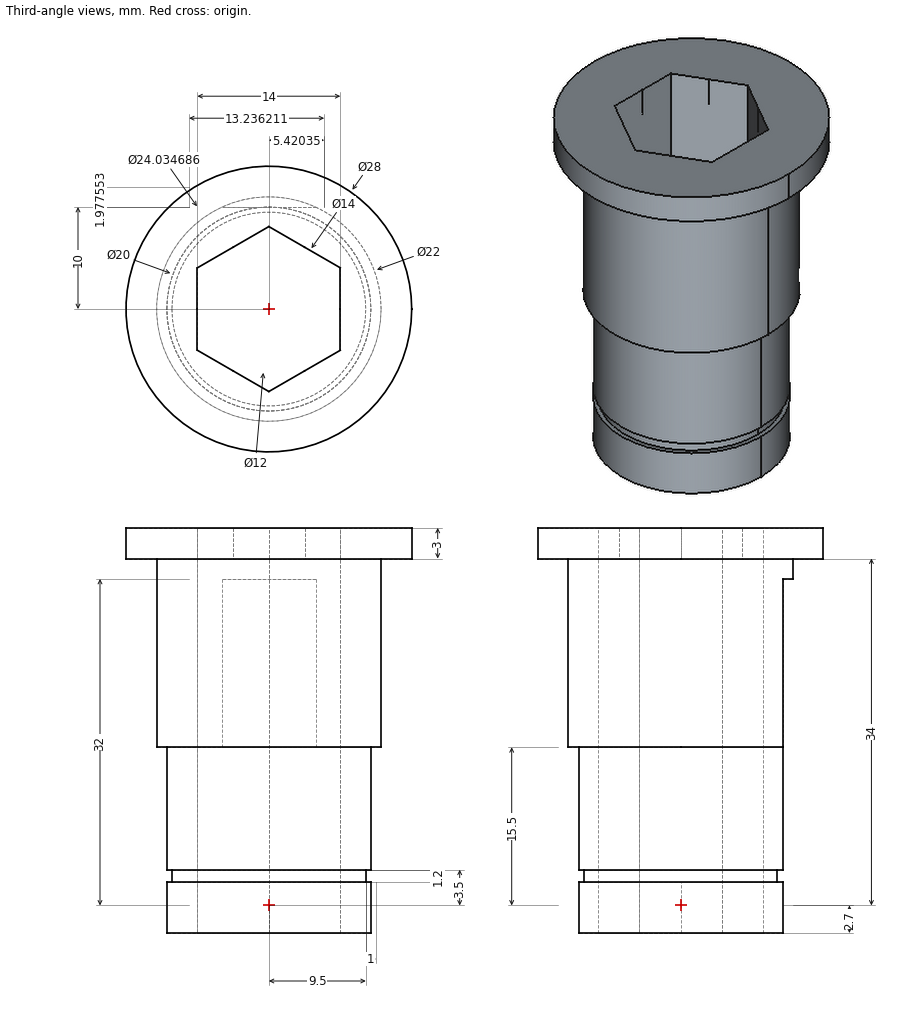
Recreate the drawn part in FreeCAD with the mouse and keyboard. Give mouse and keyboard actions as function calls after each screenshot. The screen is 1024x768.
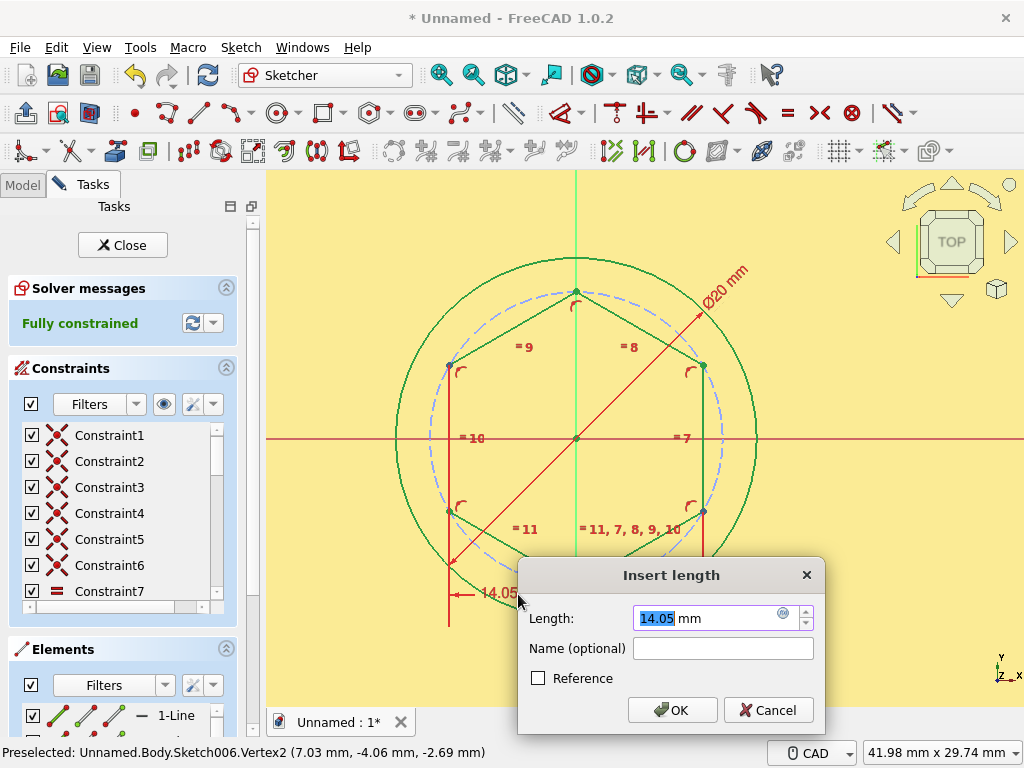
text(14)
key(Return)
key(Escape)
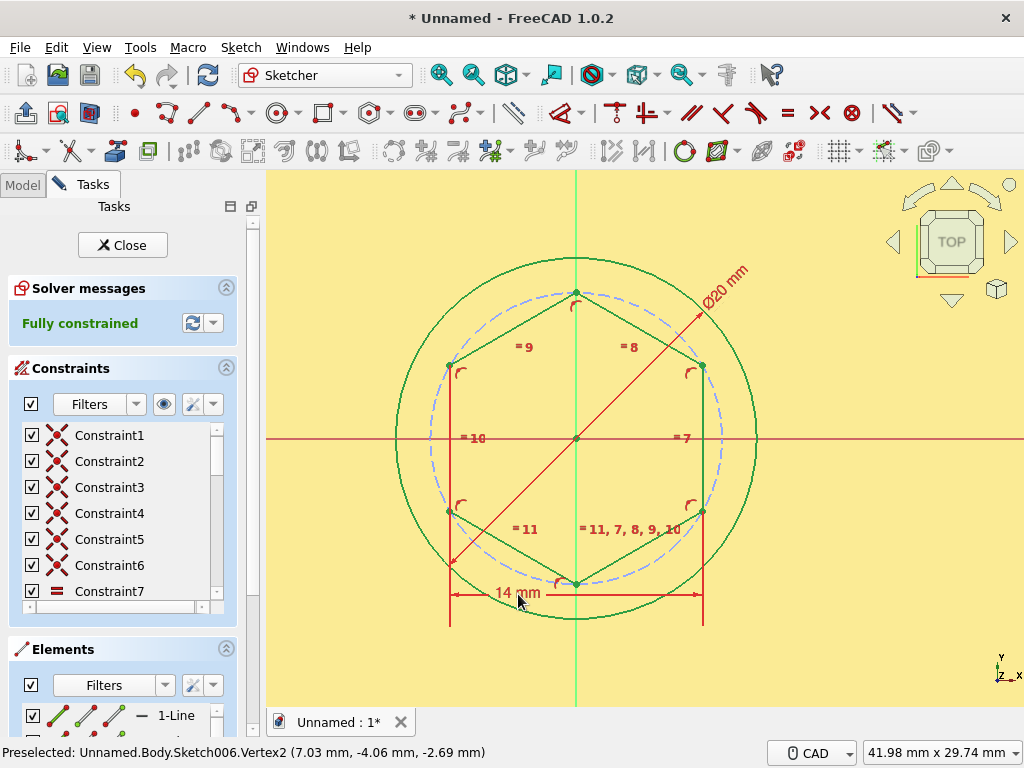
click(123, 245)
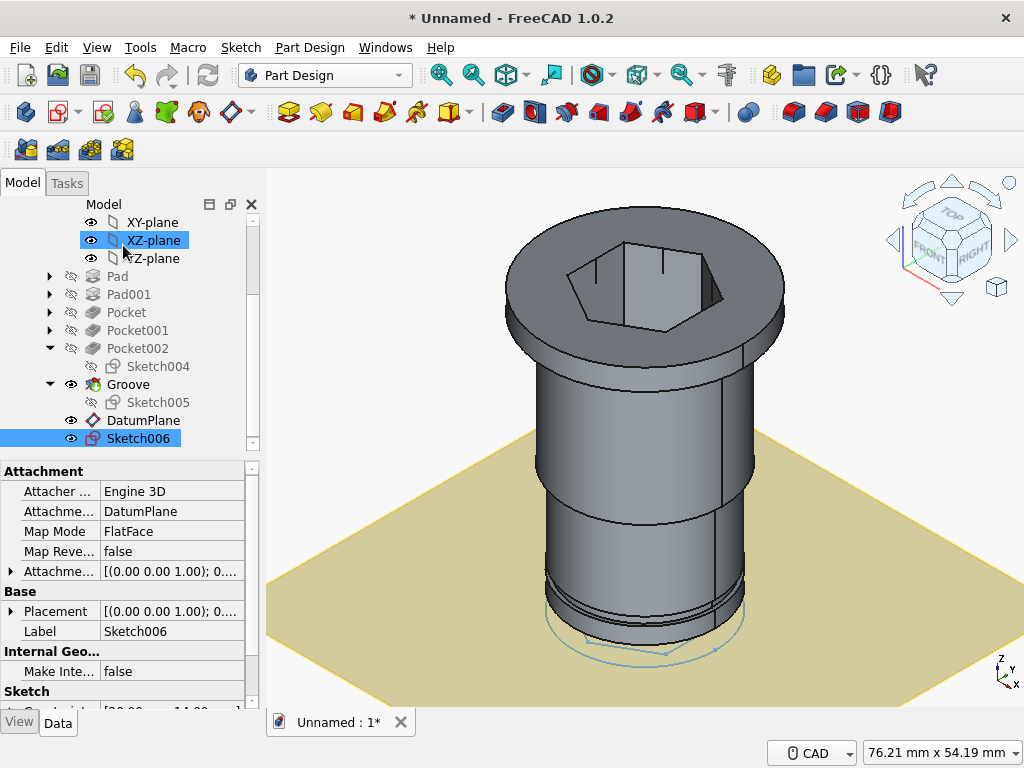
click(290, 112)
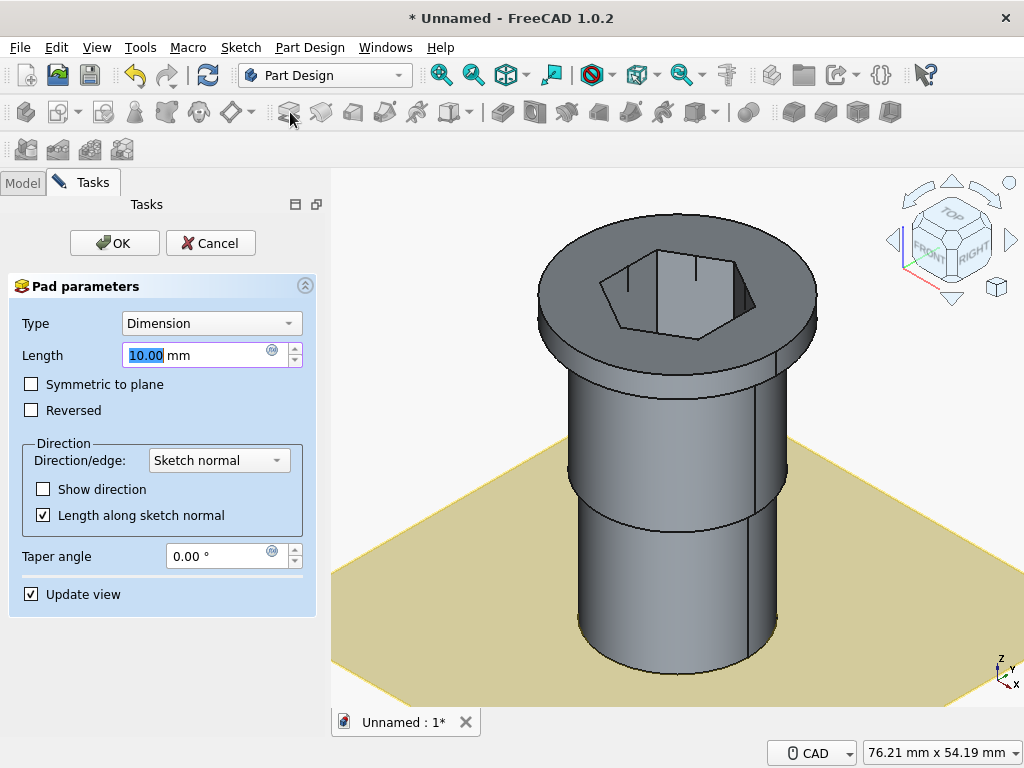
text(2.7)
key(Tab)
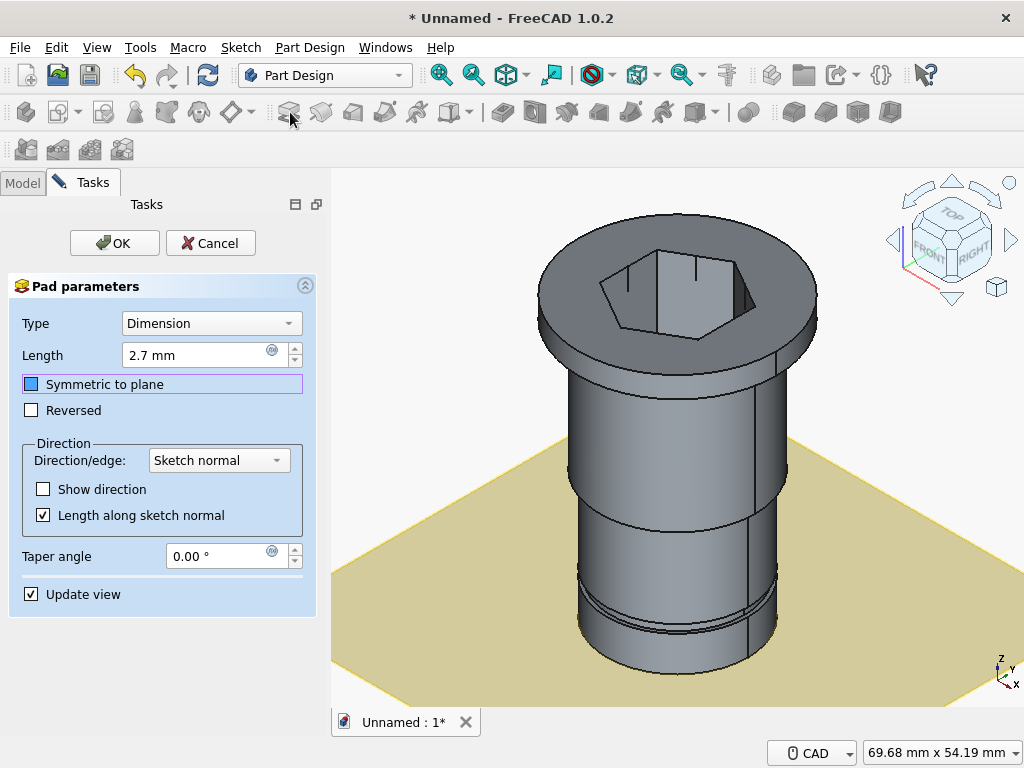
click(115, 243)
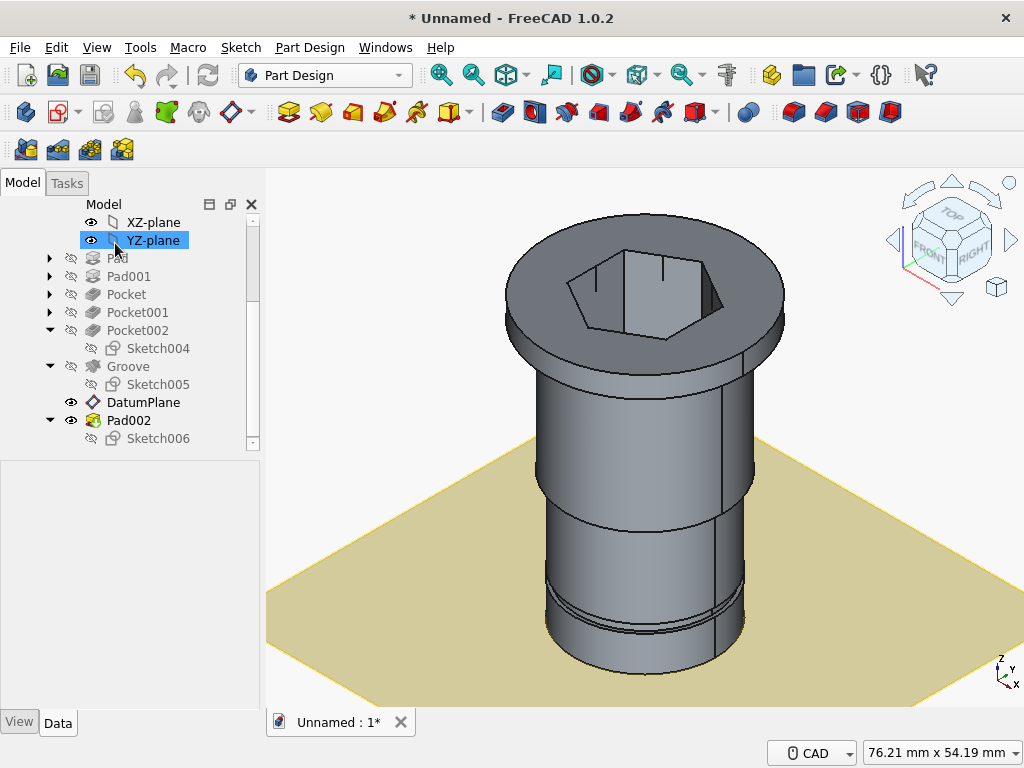
click(116, 402)
key(space)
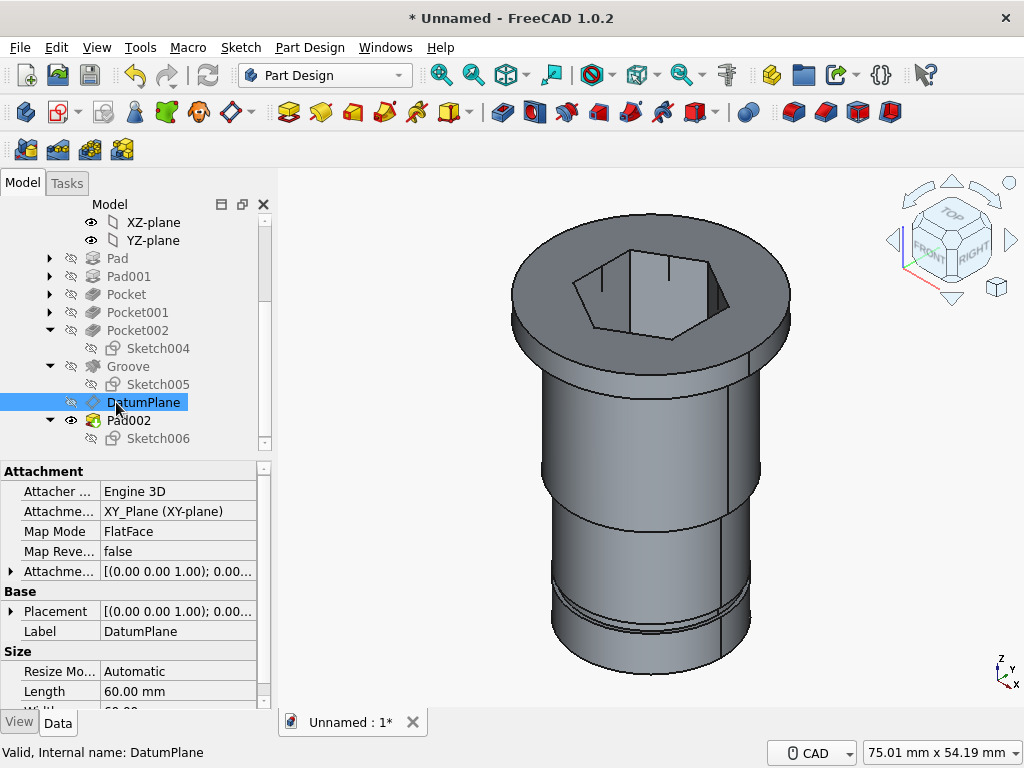
click(442, 76)